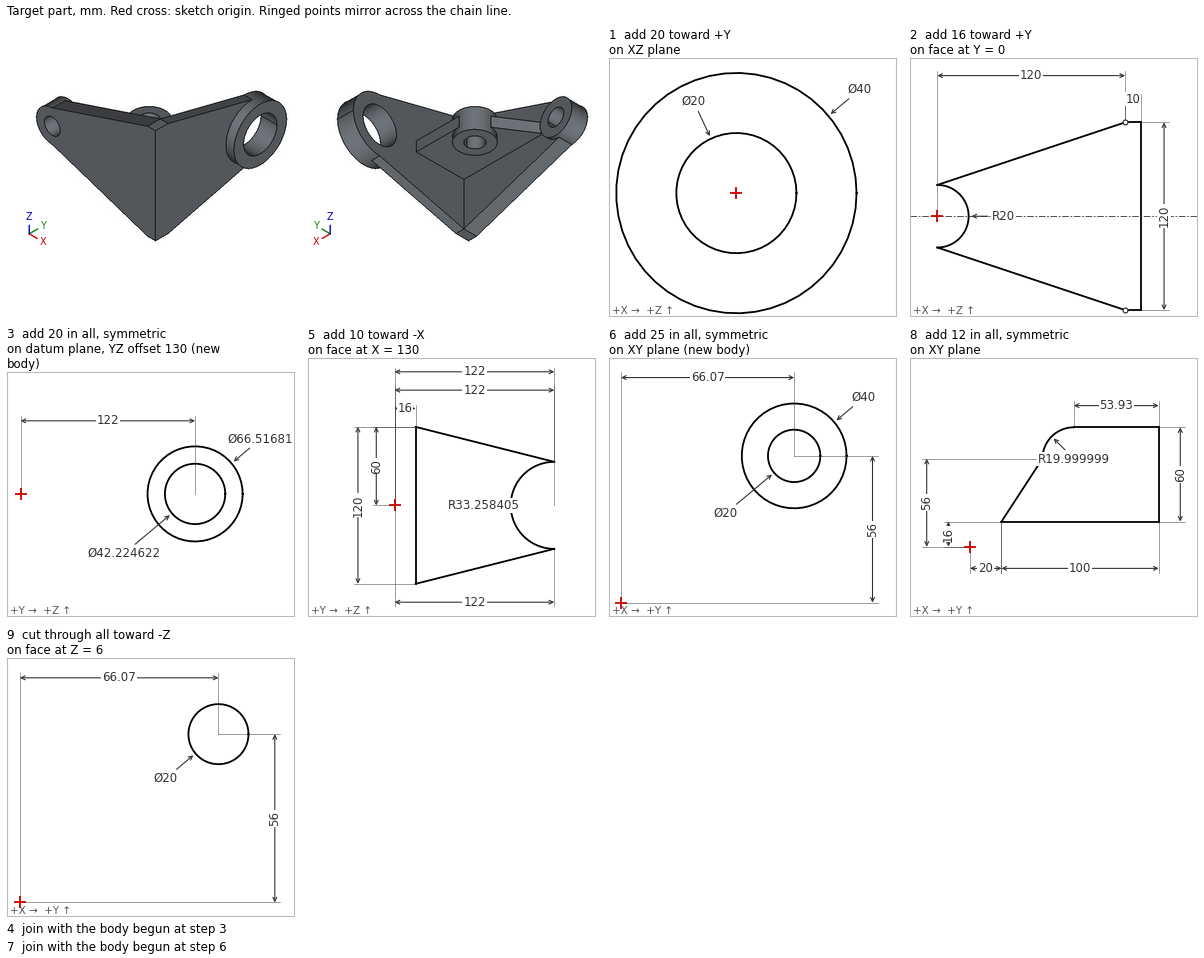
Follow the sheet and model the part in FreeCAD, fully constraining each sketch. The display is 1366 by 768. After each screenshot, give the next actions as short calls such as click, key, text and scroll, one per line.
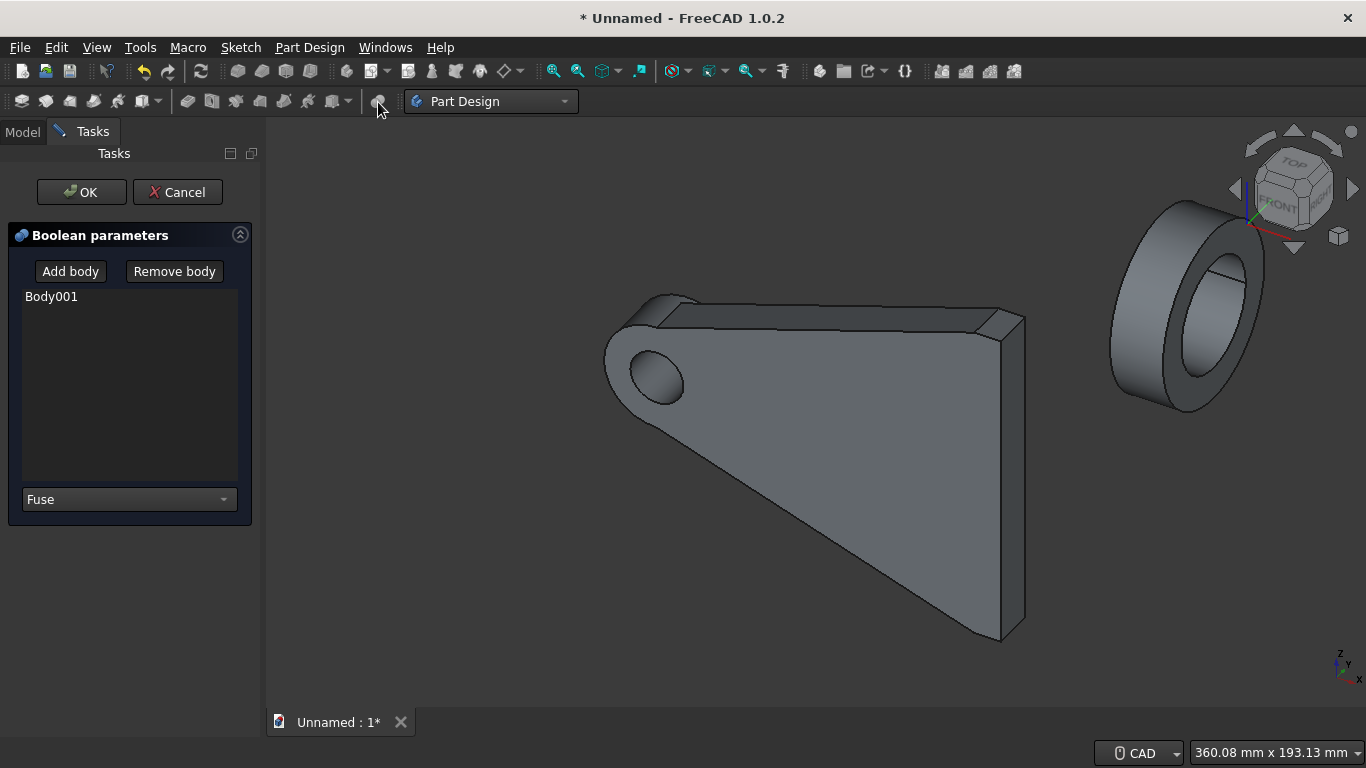
click(82, 192)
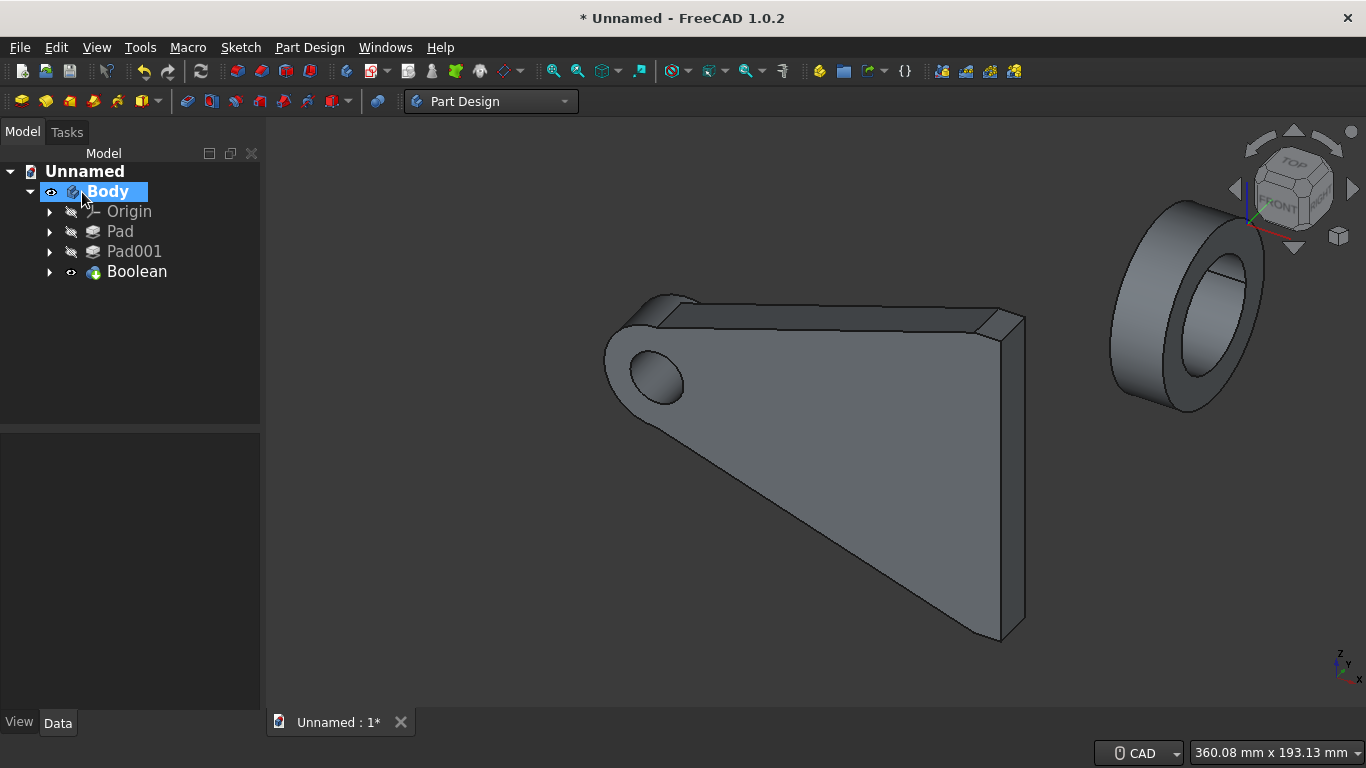
click(554, 72)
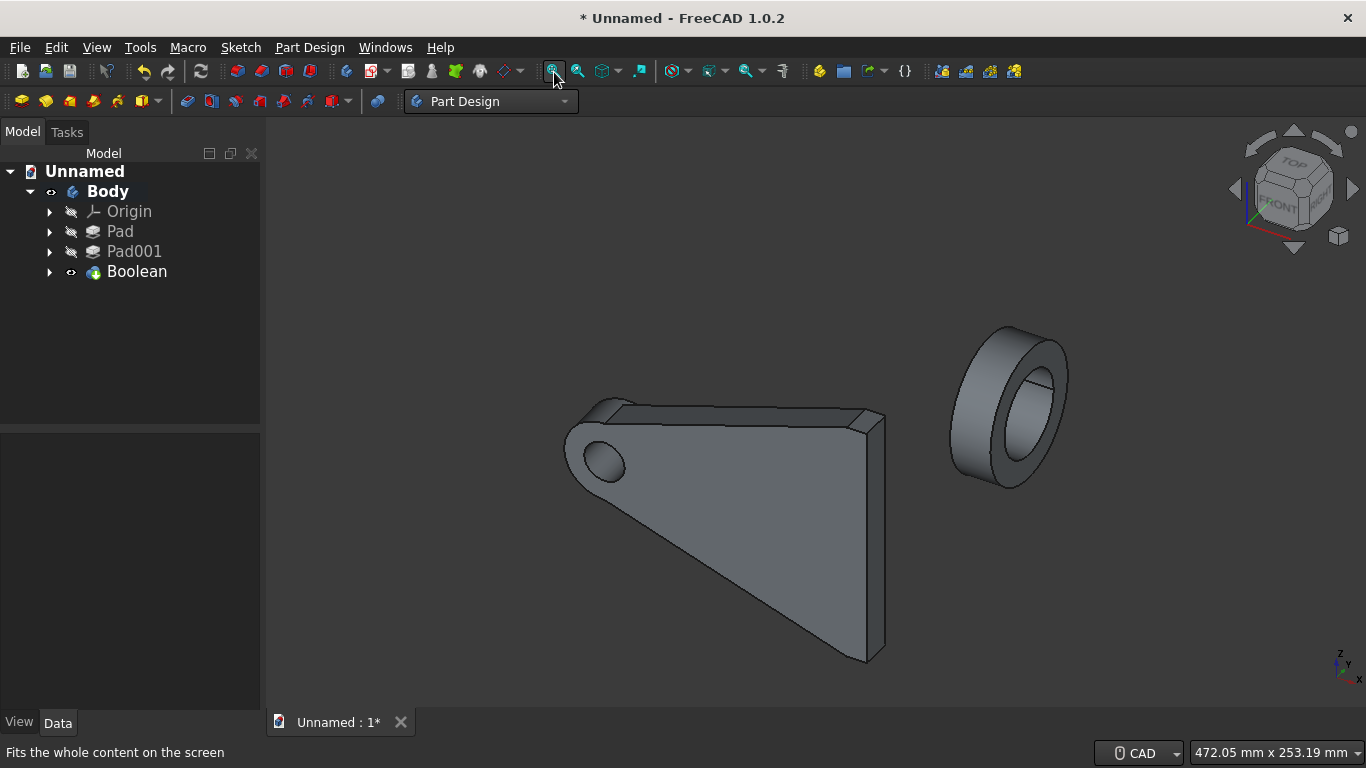
click(876, 473)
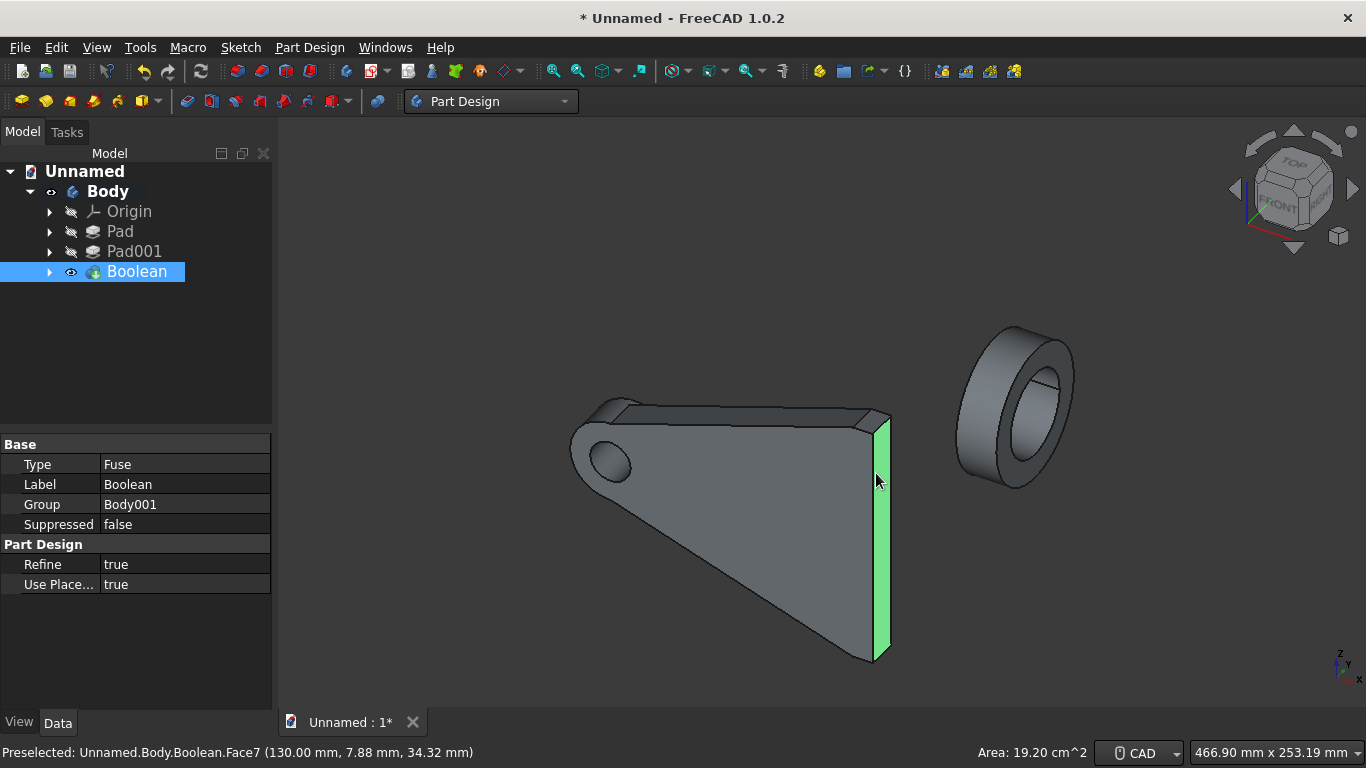
click(372, 72)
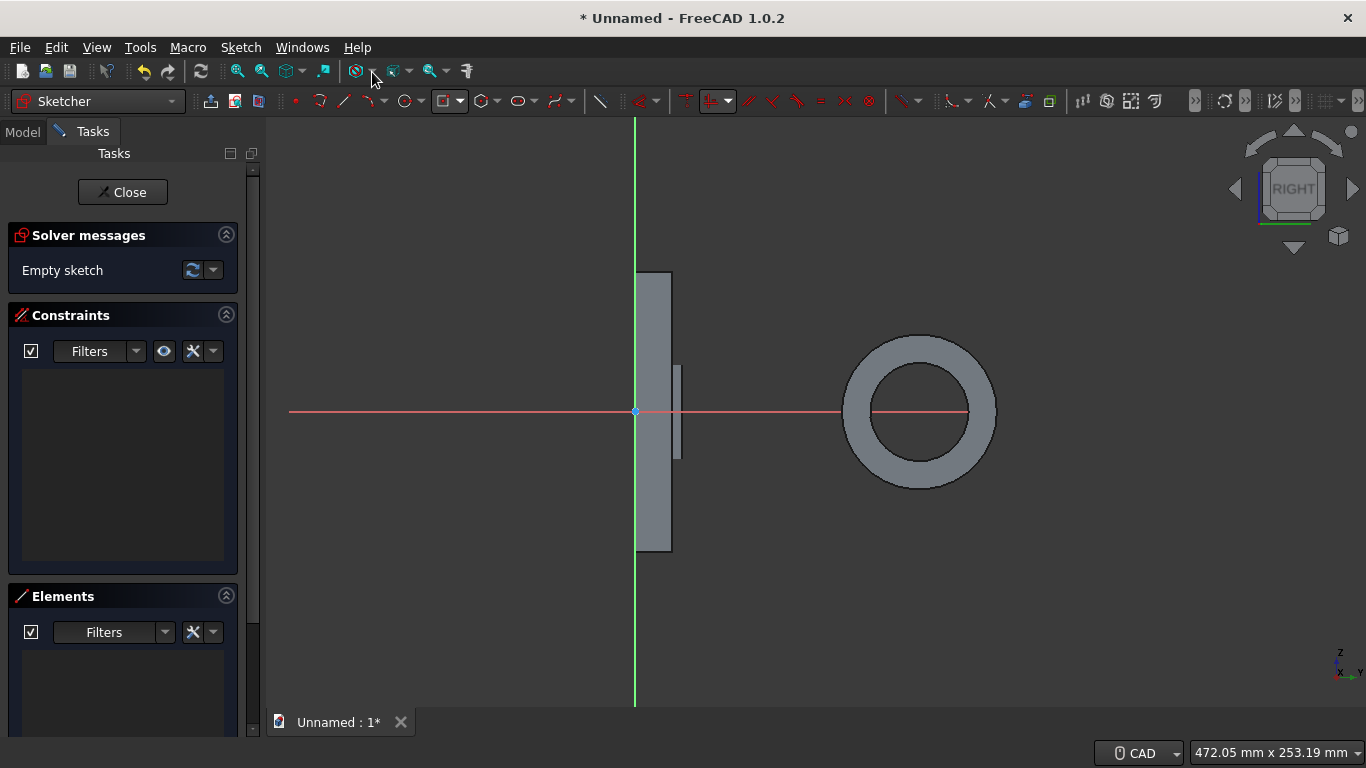
click(260, 102)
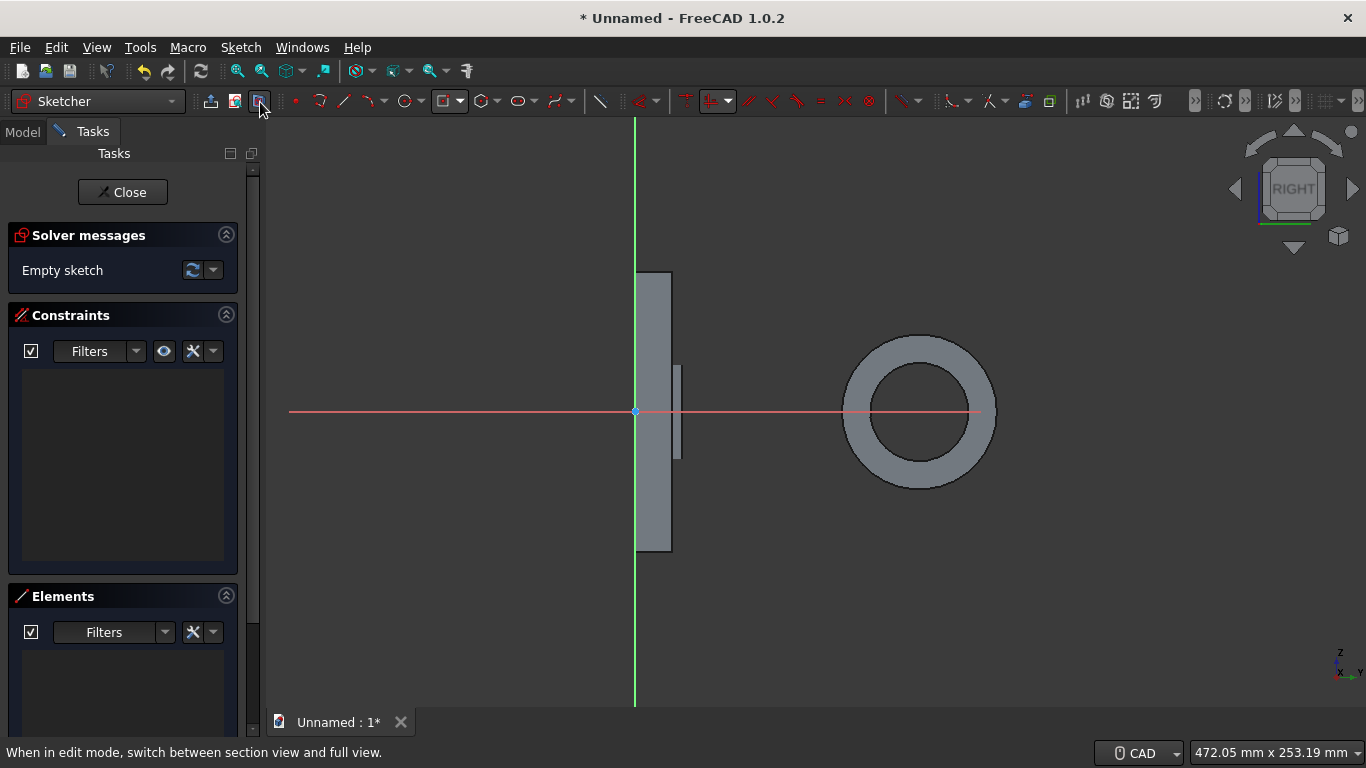
key(g)
key(m)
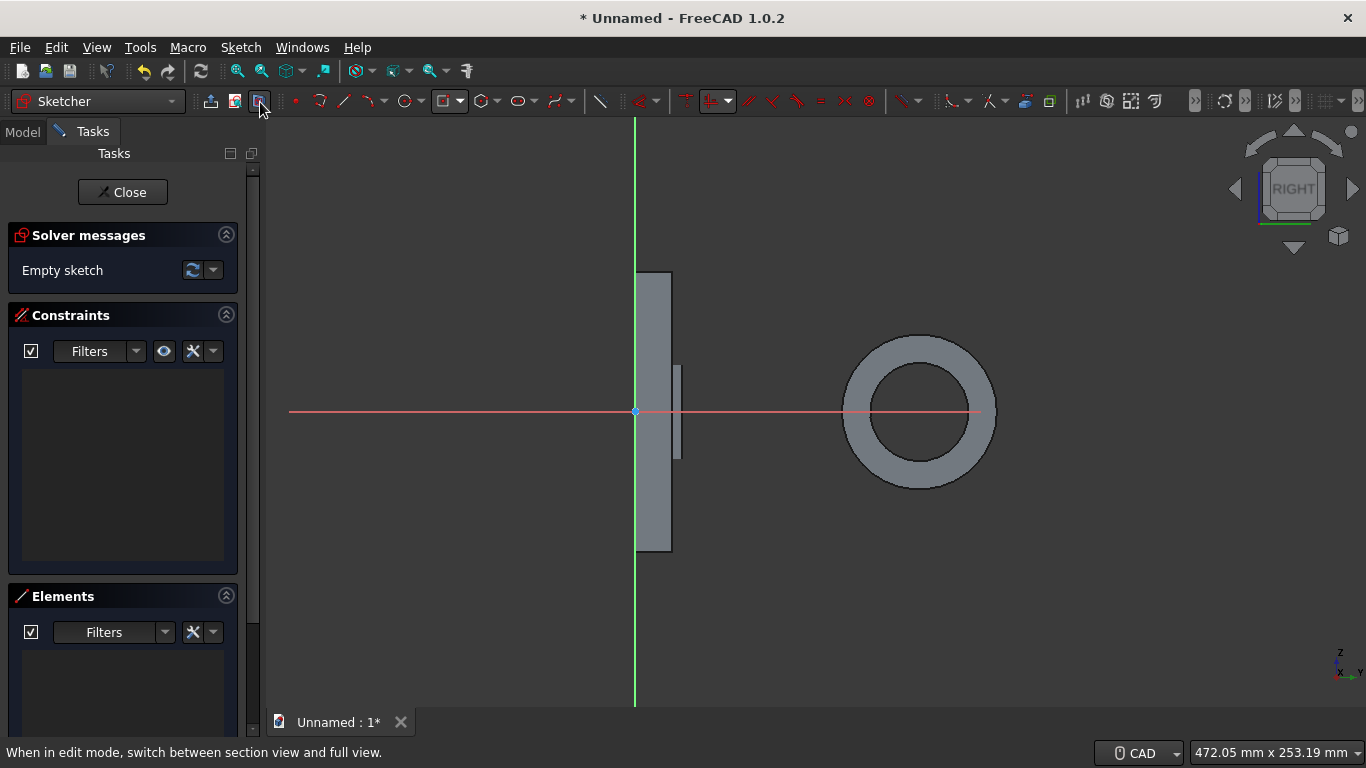
click(919, 334)
click(672, 272)
click(672, 552)
click(919, 490)
right_click(919, 490)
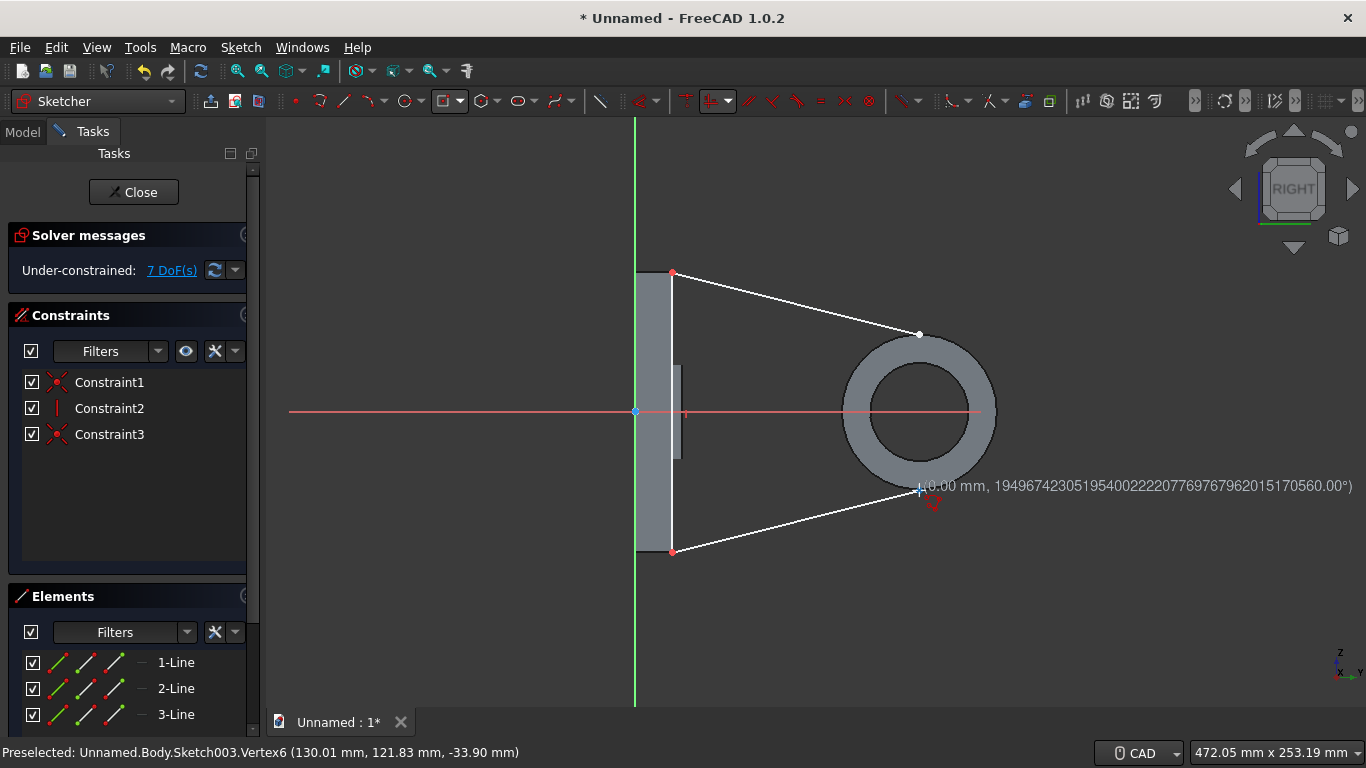
key(g)
key(3)
key(a)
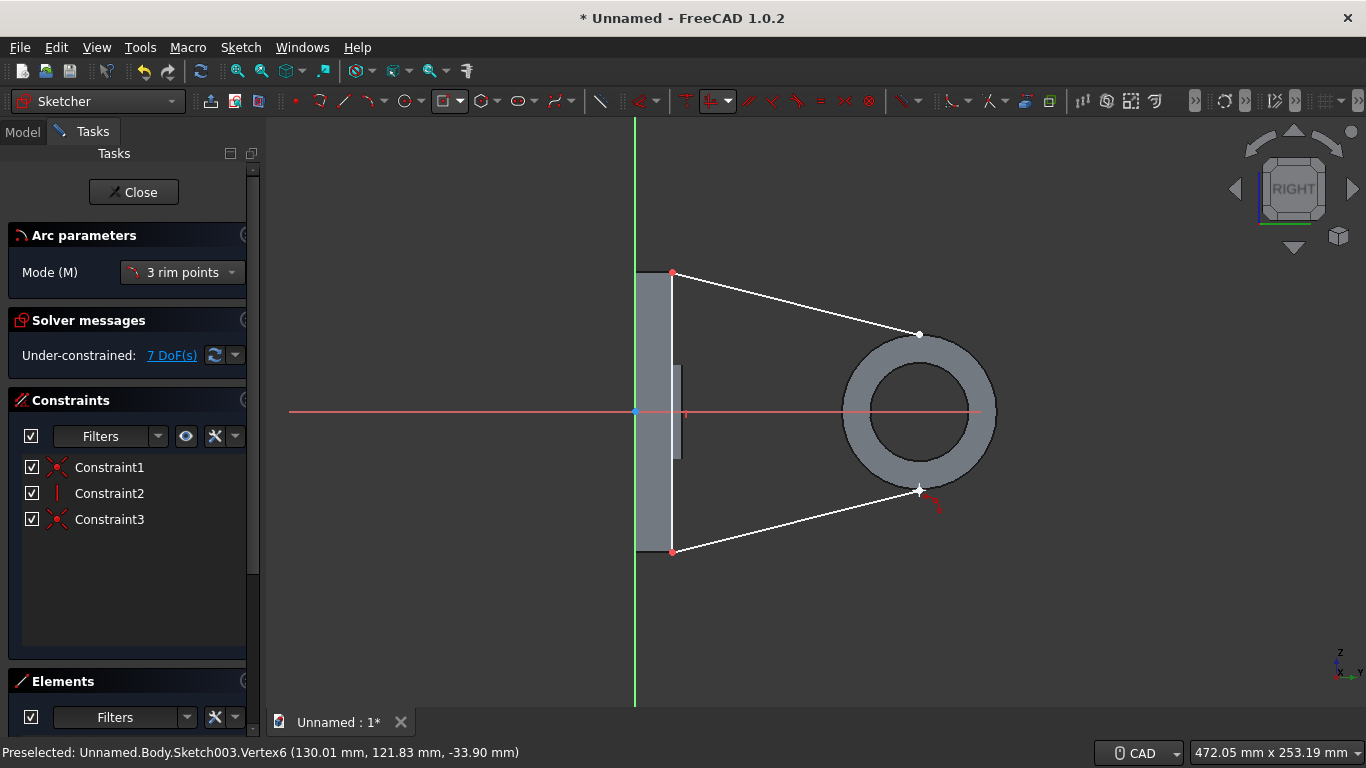
click(919, 491)
click(919, 335)
click(846, 388)
key(Escape)